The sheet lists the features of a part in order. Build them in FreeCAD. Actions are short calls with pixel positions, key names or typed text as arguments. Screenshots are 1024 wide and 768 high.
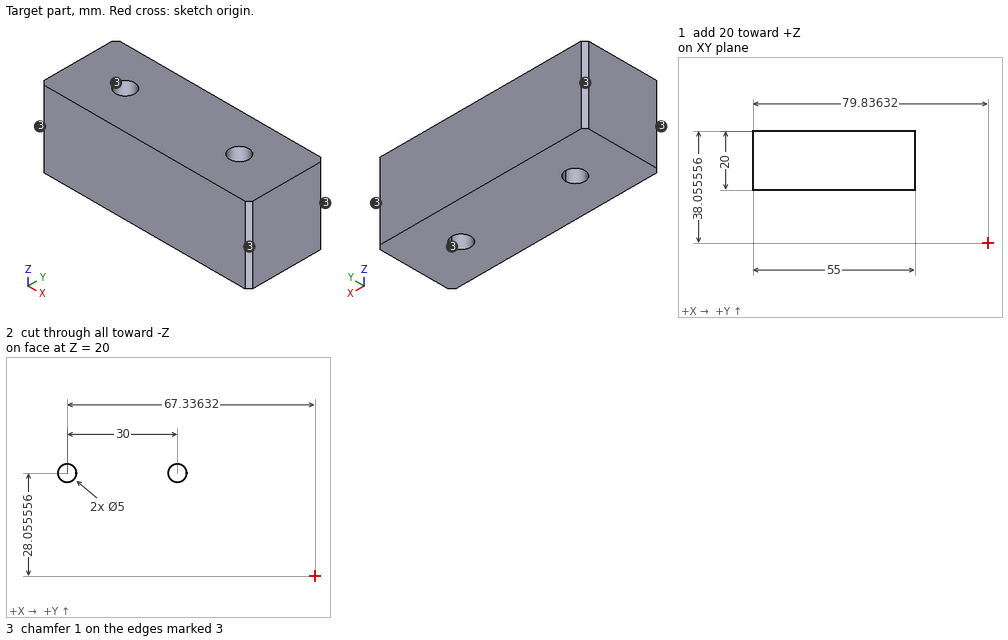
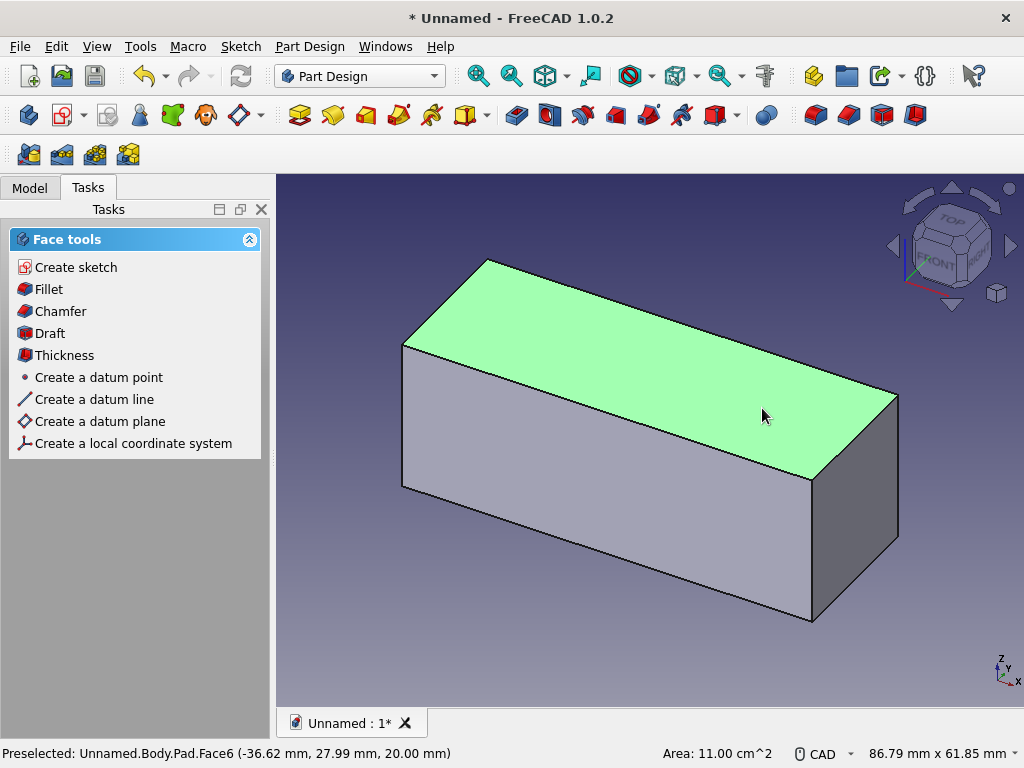
click(62, 116)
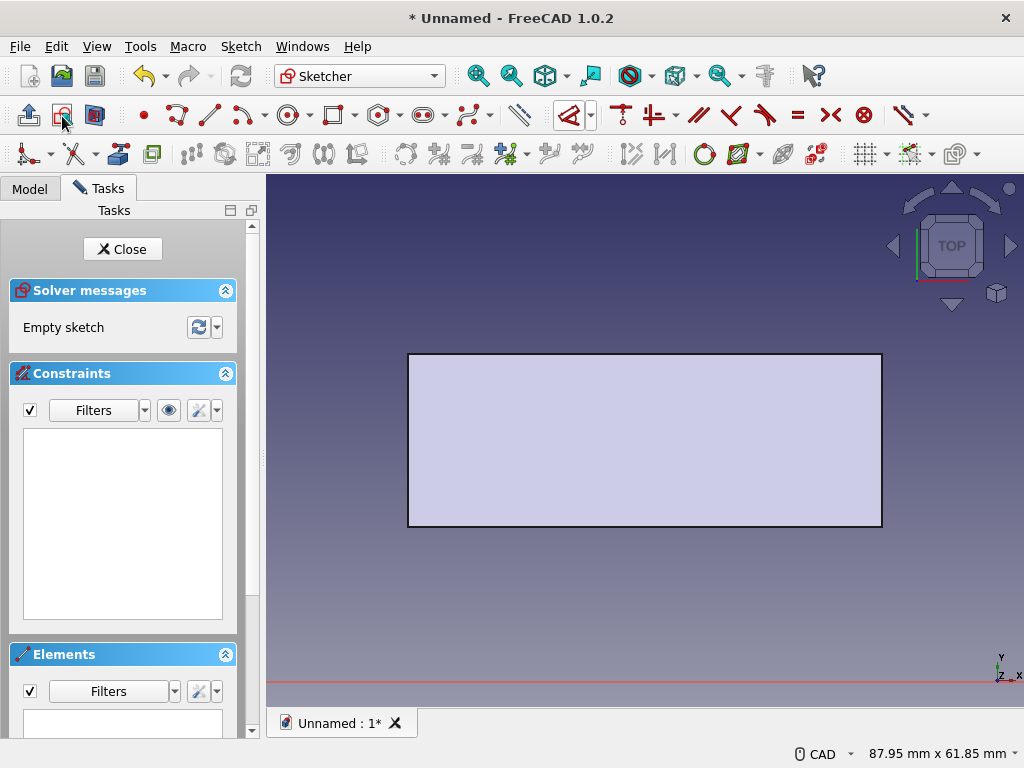
scroll(294, 217, down, 2)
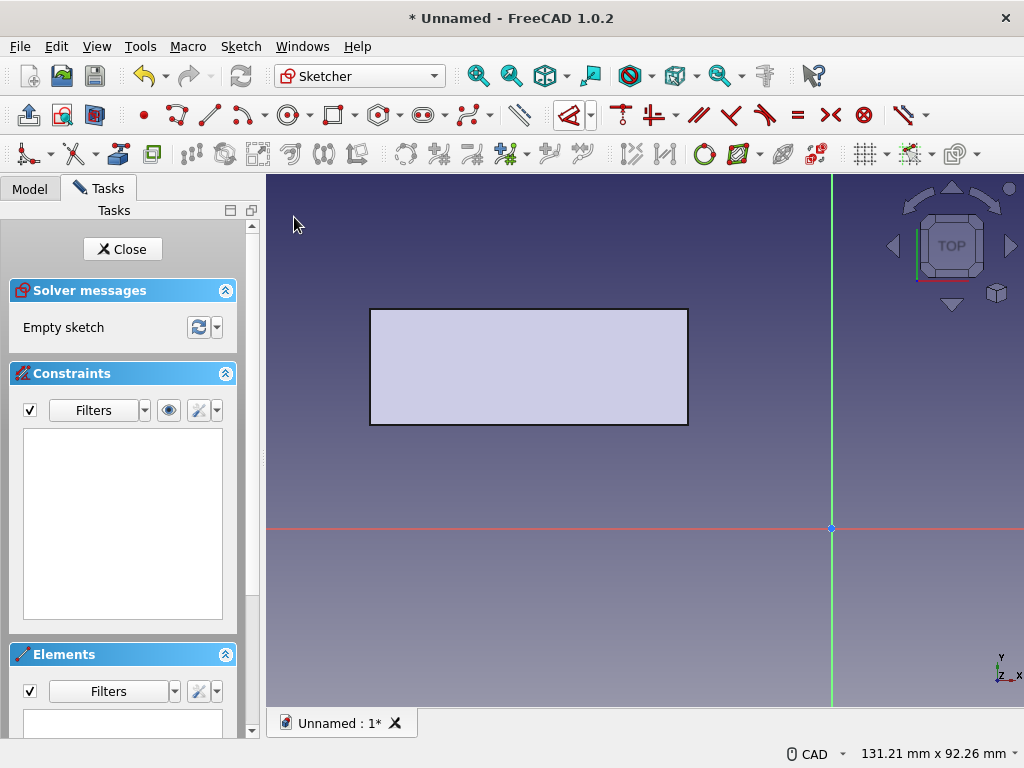
click(288, 116)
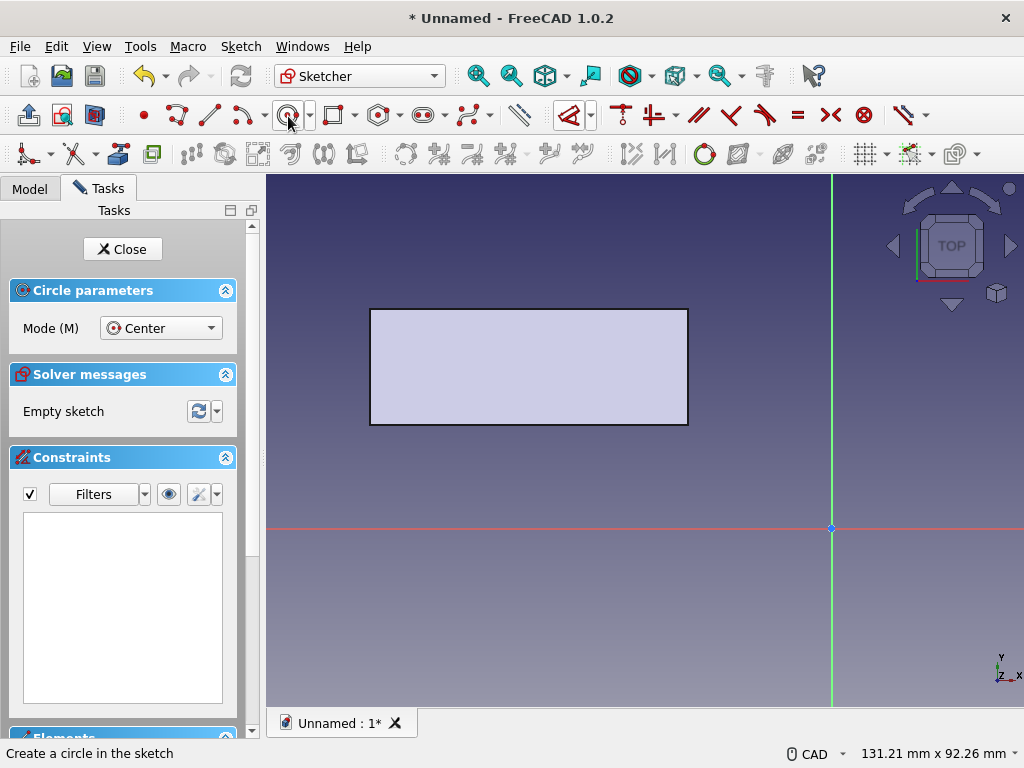
scroll(443, 367, up, 3)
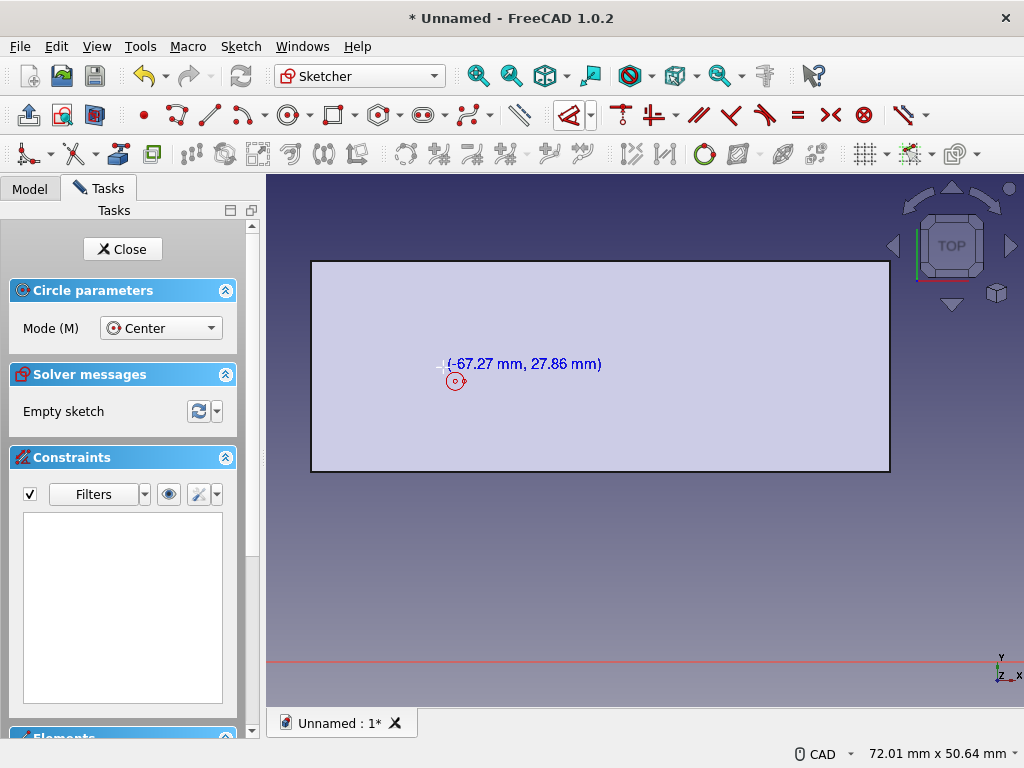
click(442, 366)
click(461, 348)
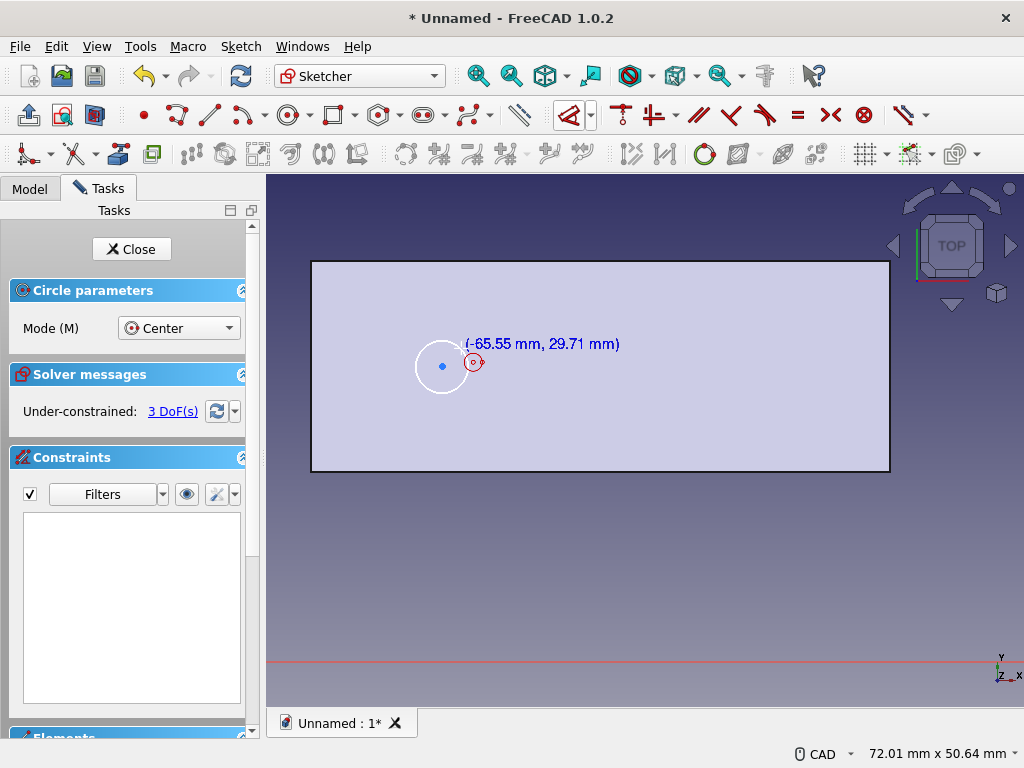
click(758, 366)
click(777, 348)
key(Escape)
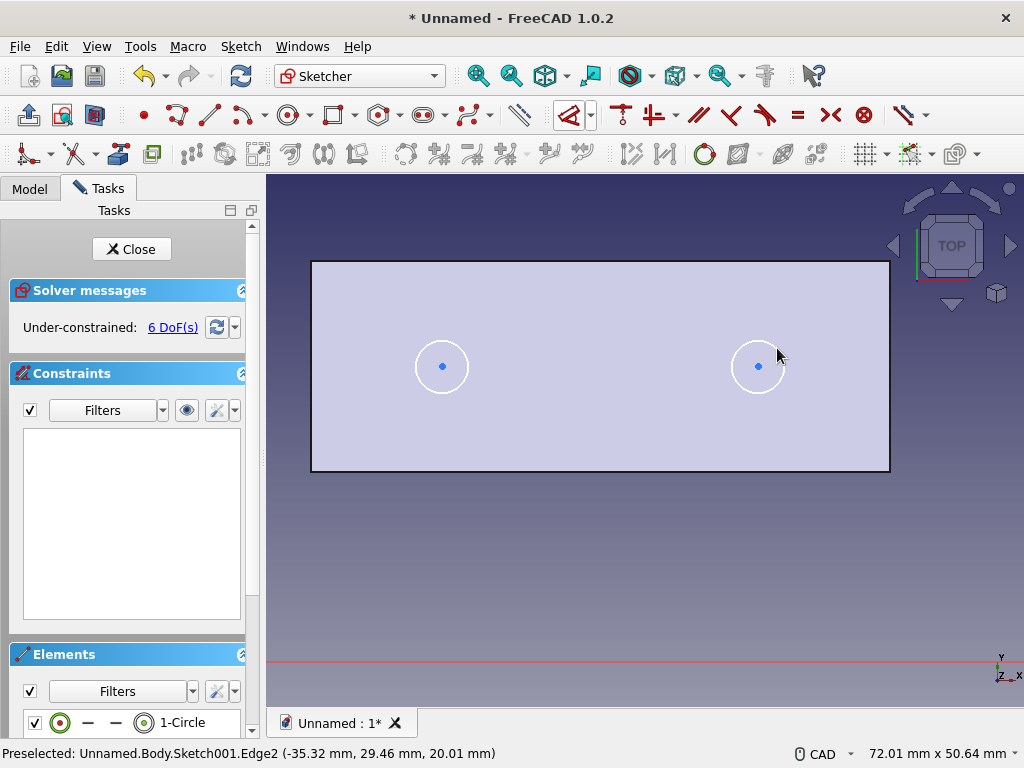
click(460, 348)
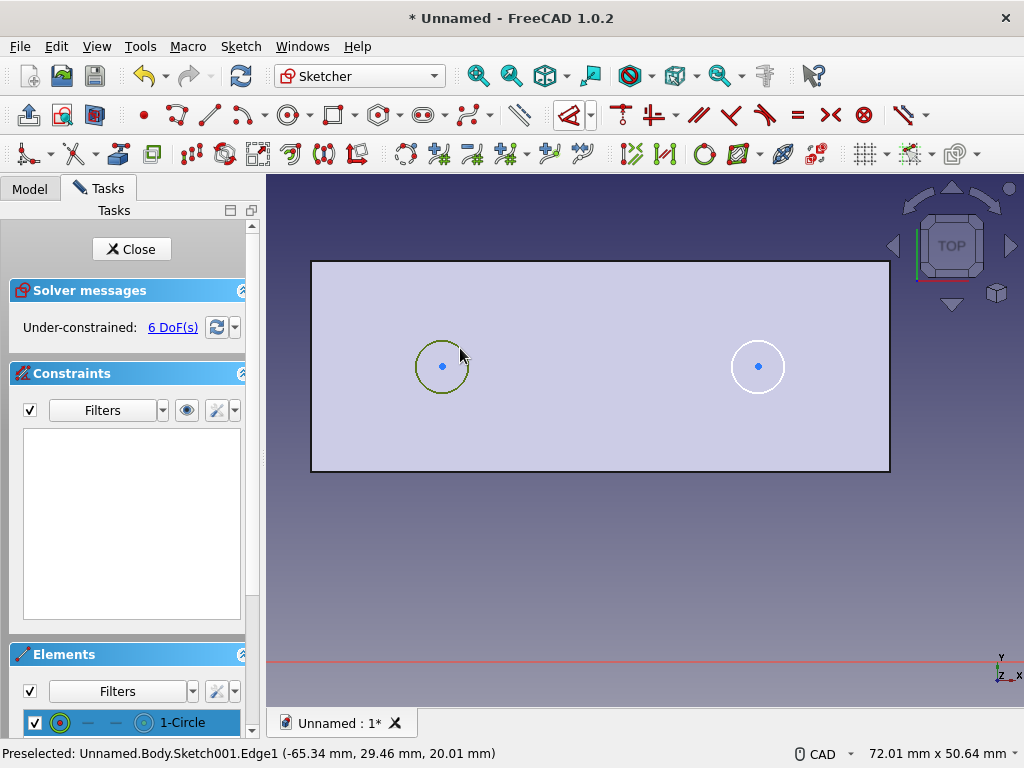
click(776, 348)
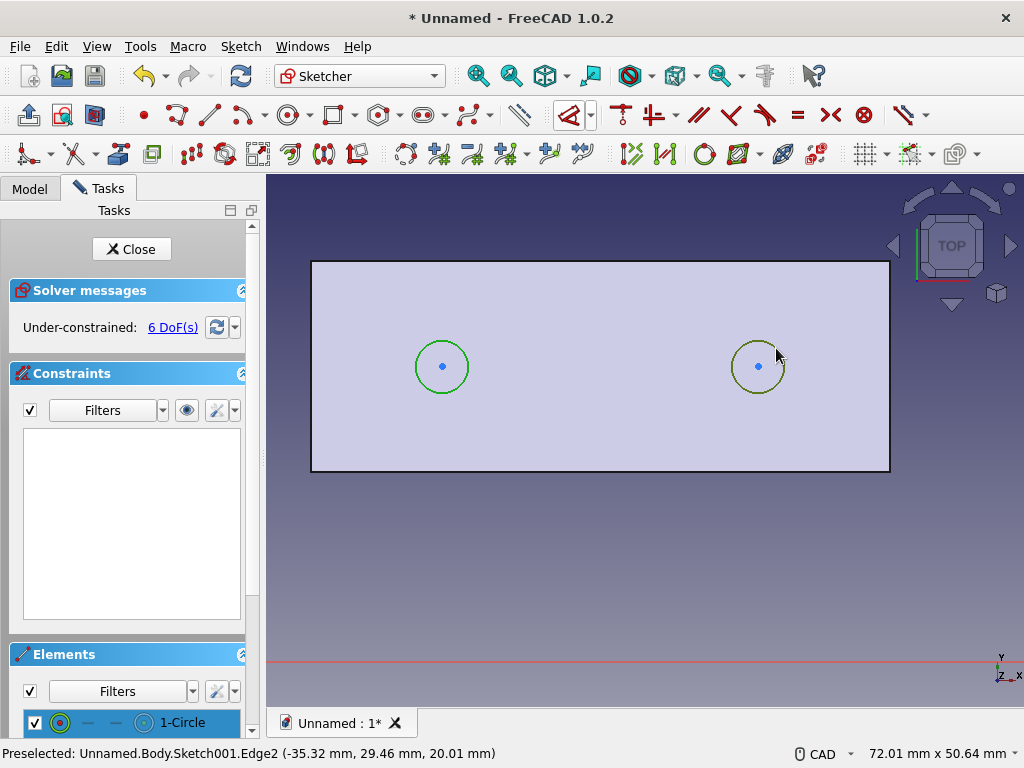
click(798, 116)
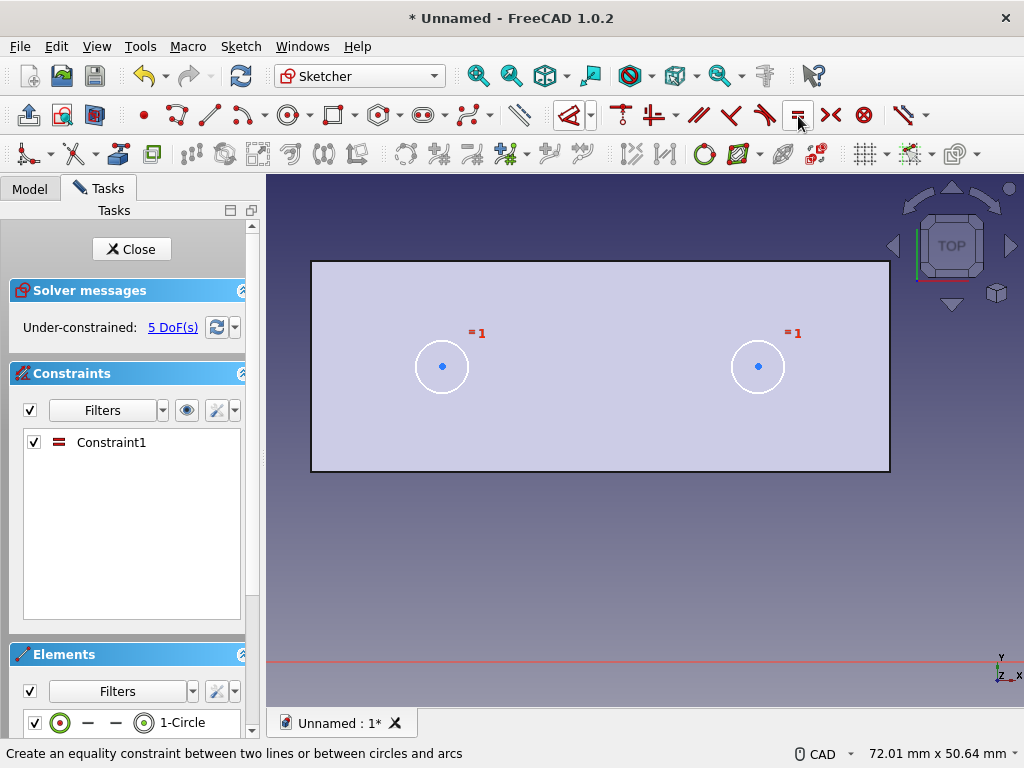
click(442, 367)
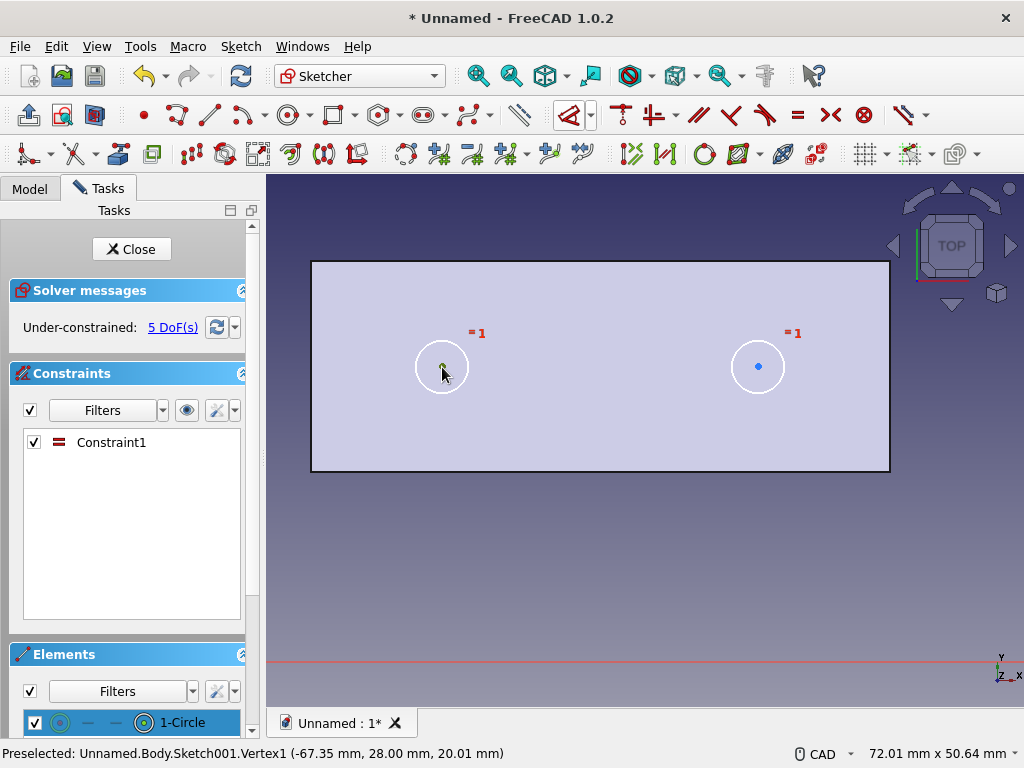
click(758, 367)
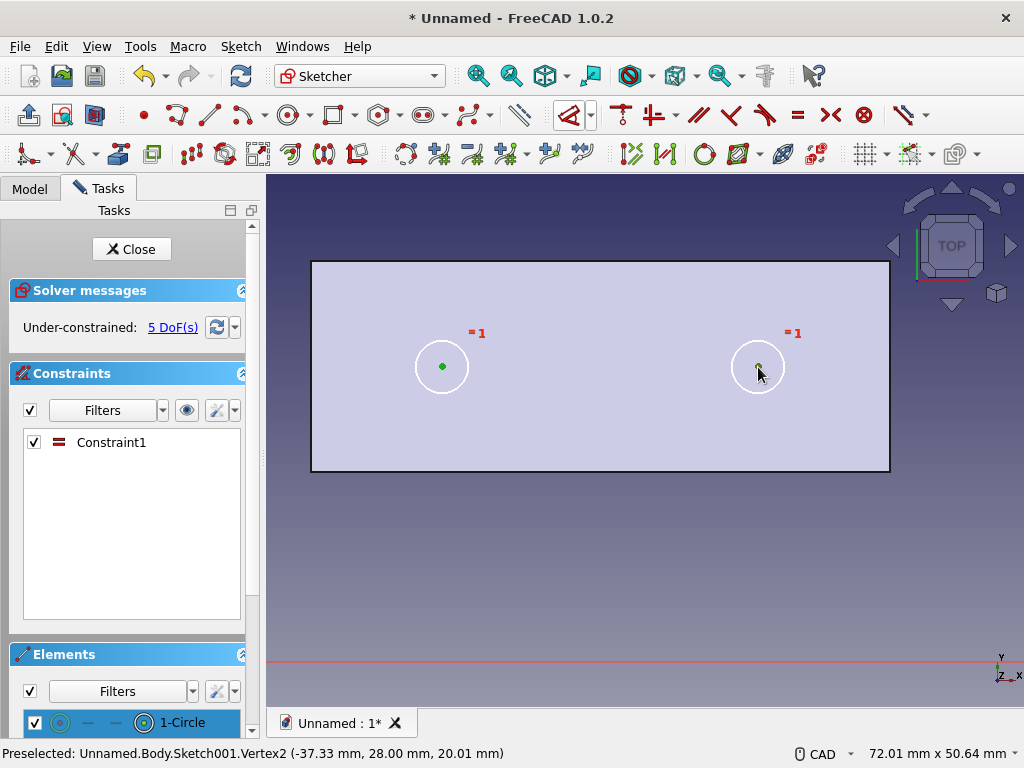
click(676, 116)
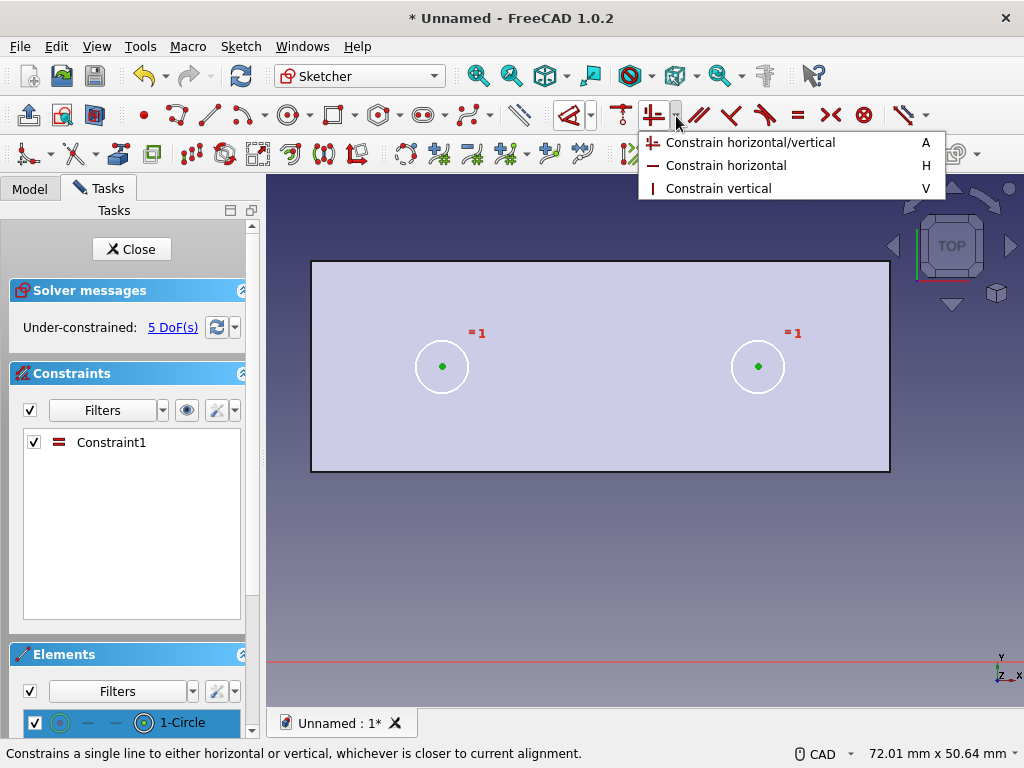
click(792, 166)